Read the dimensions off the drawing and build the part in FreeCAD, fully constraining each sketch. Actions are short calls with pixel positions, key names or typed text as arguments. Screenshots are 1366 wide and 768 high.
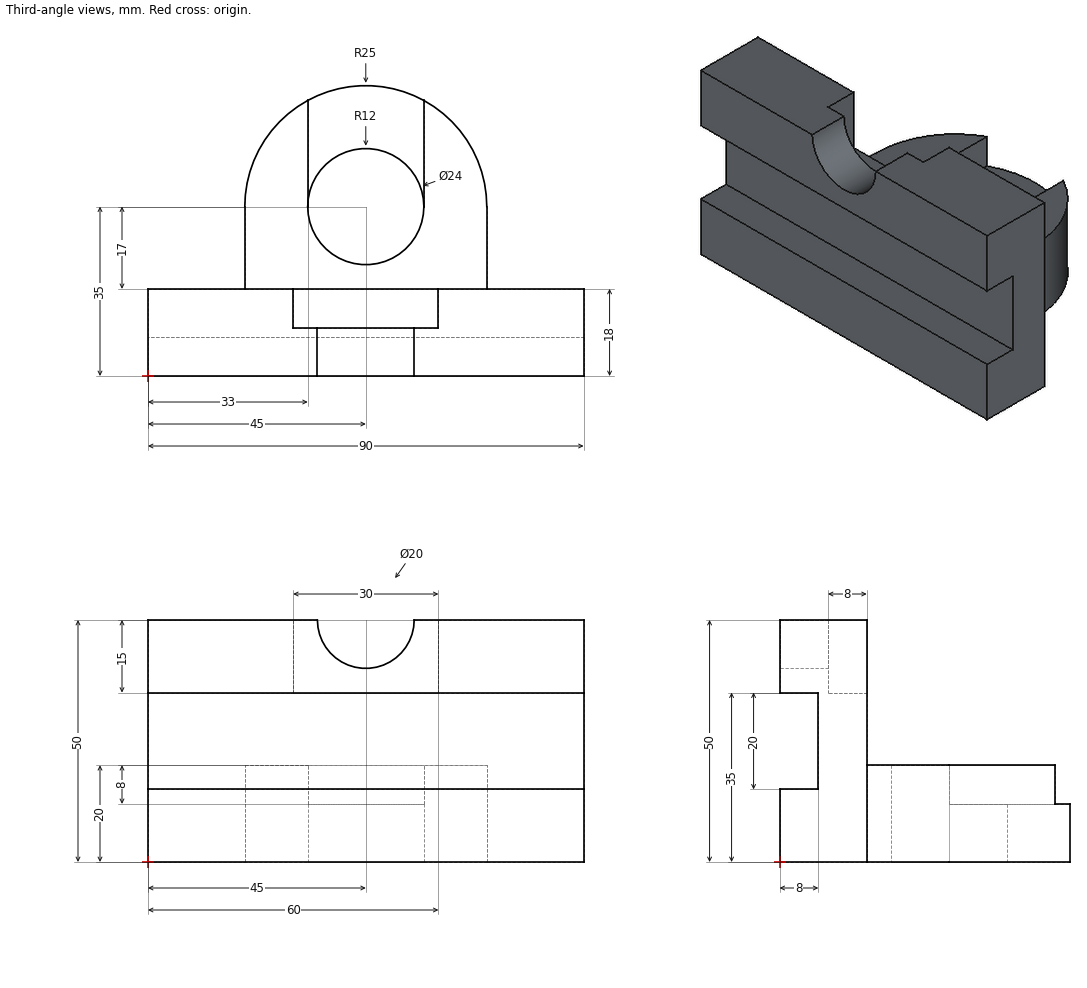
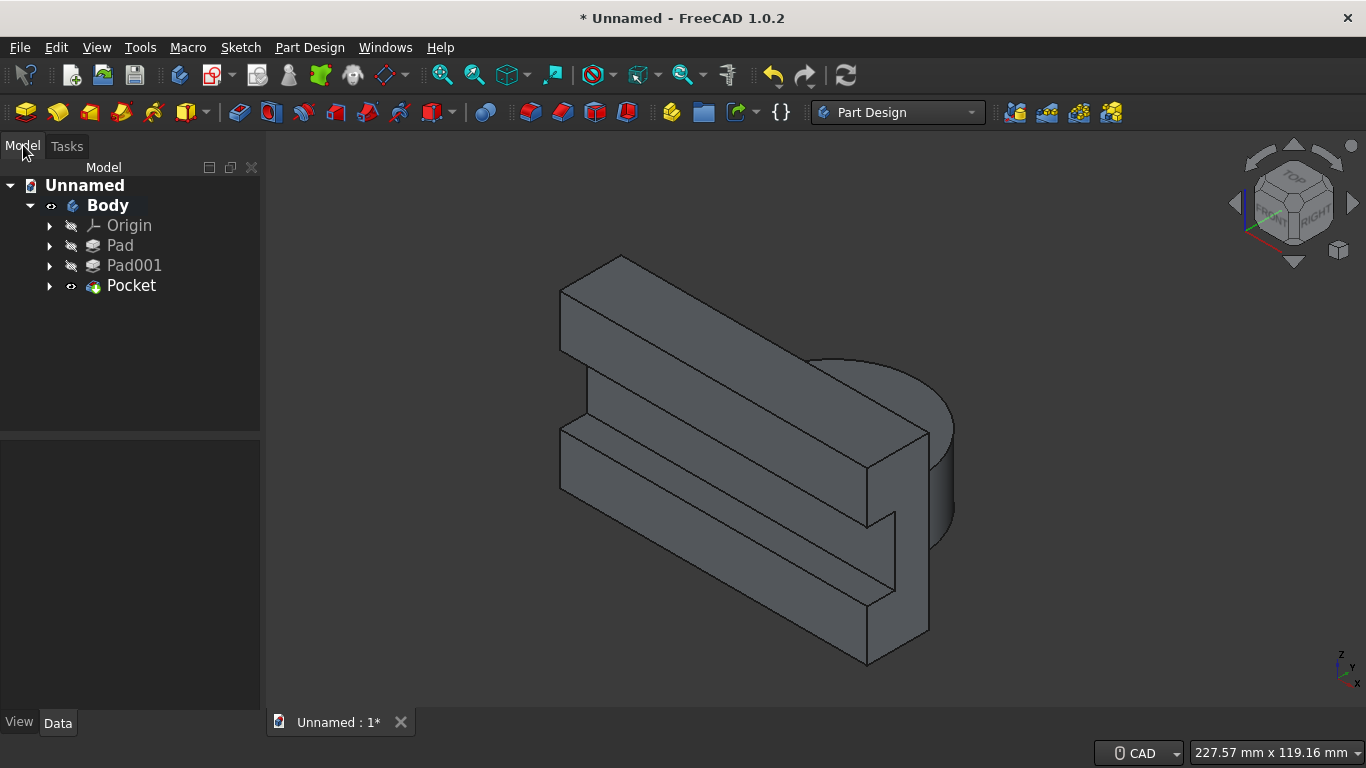
click(50, 226)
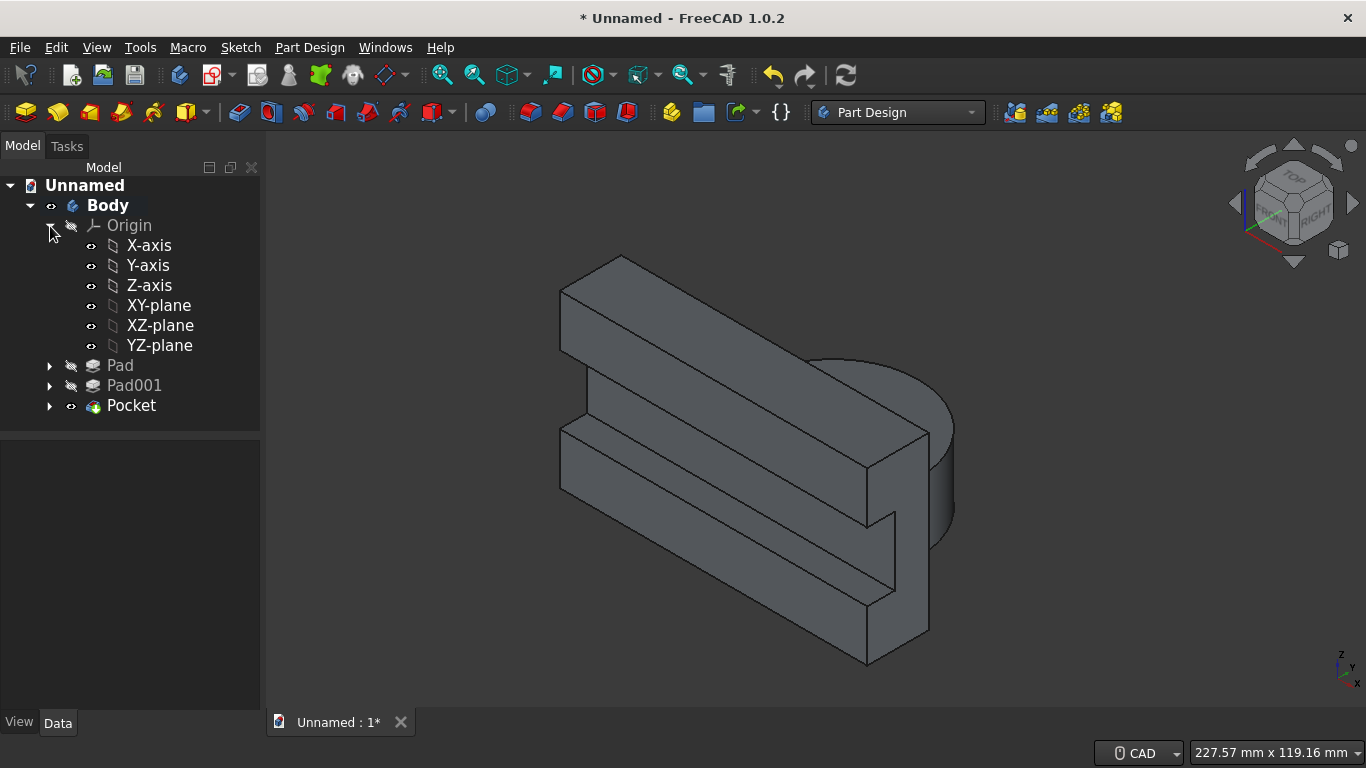
click(136, 306)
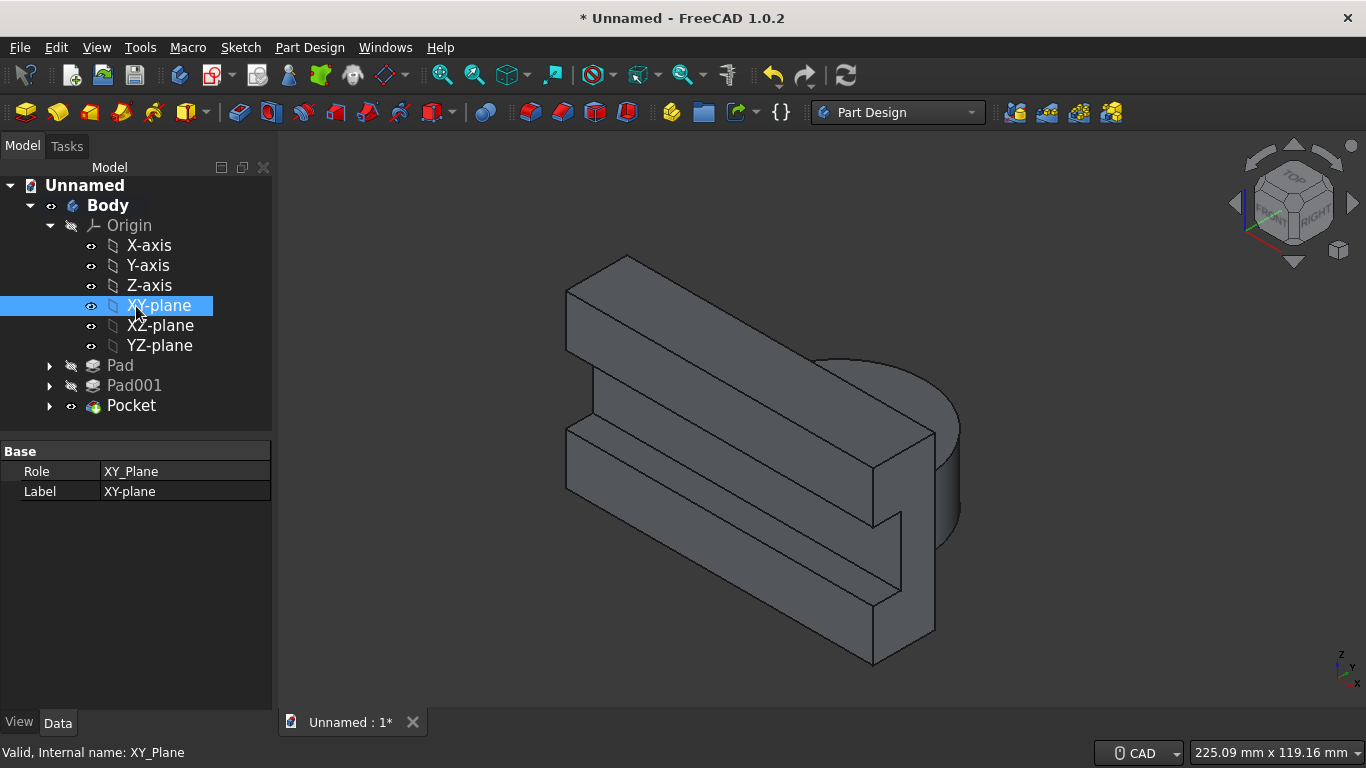
click(386, 76)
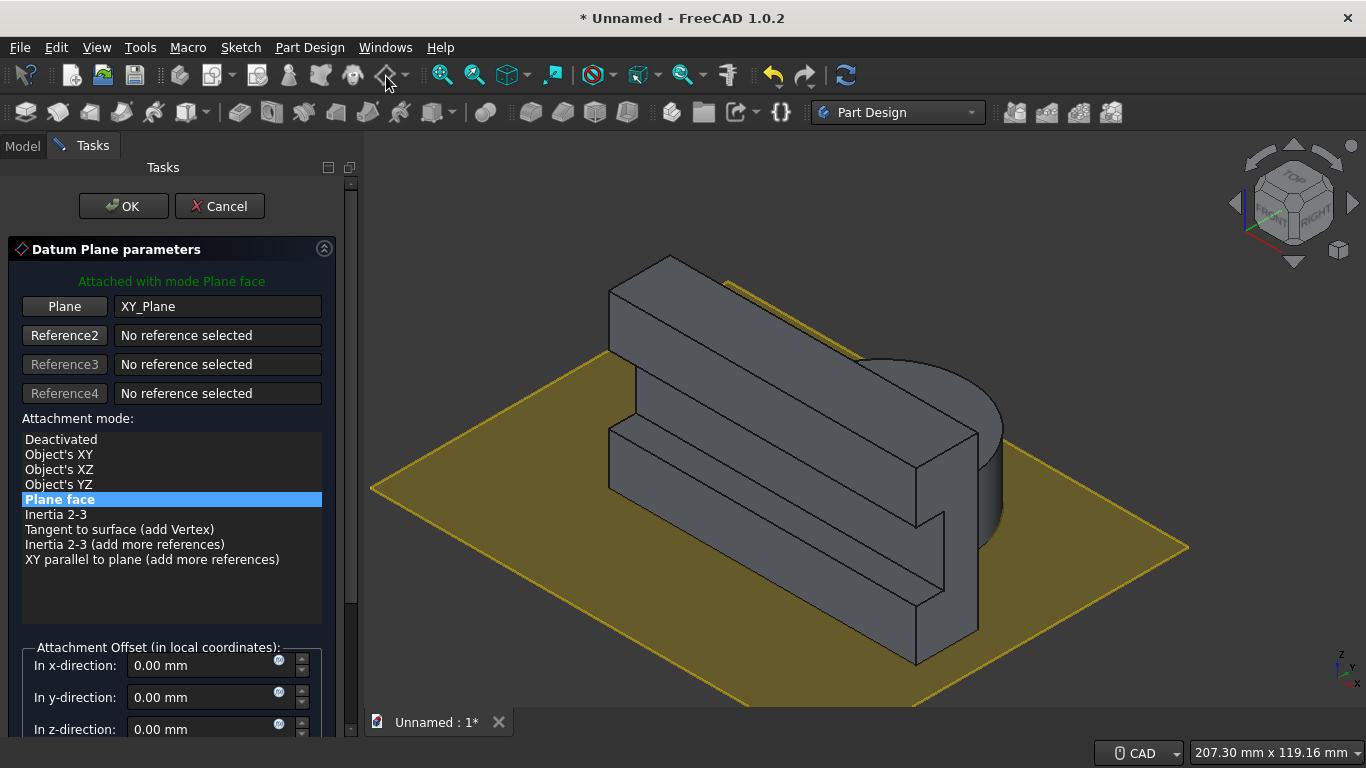
scroll(351, 456, down, 2)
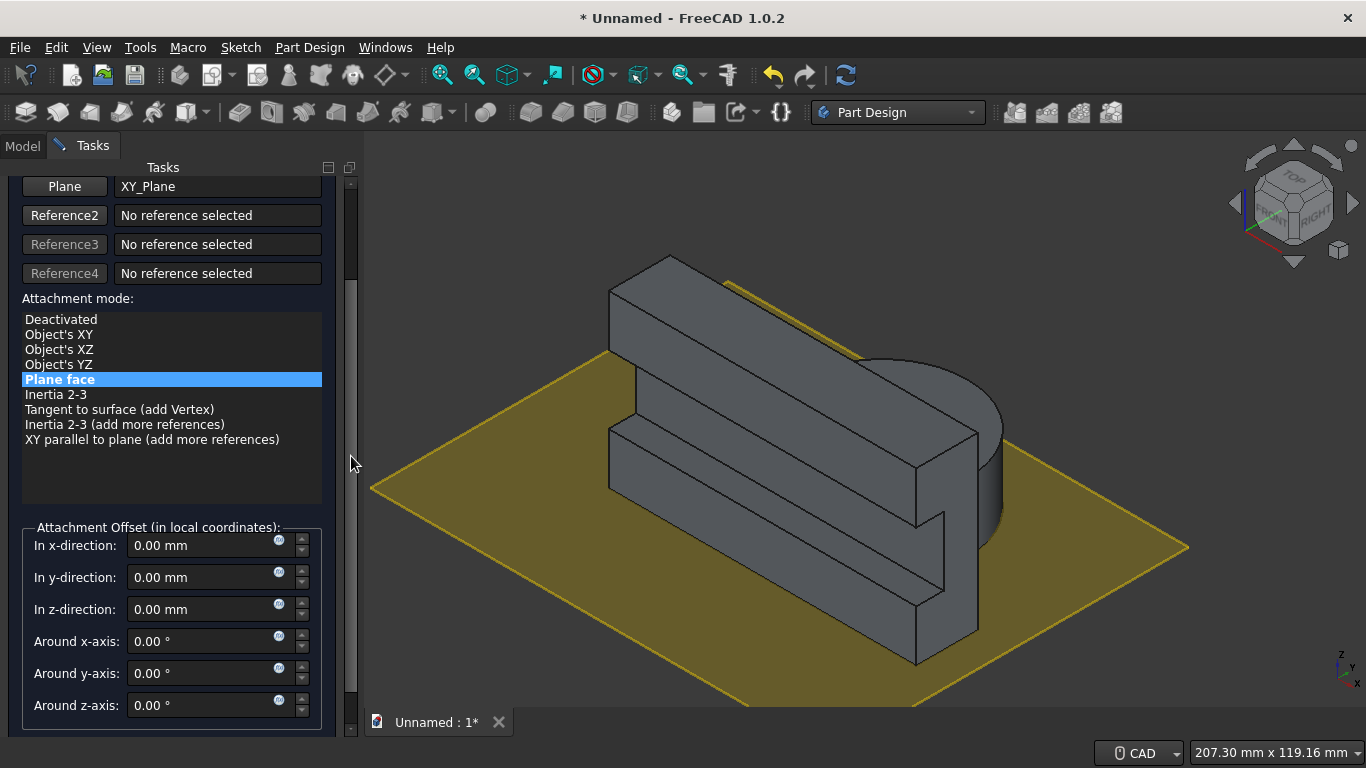
triple_click(210, 609)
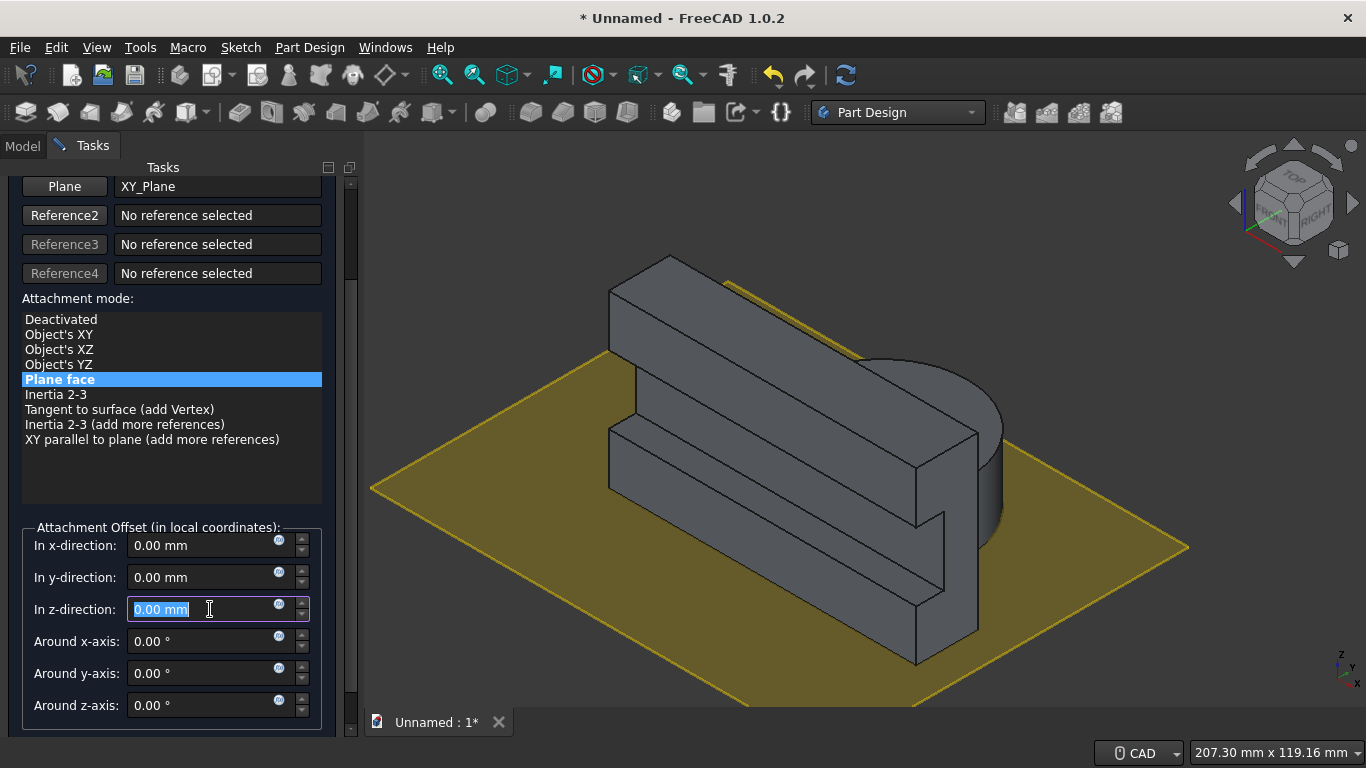
text(12)
key(Tab)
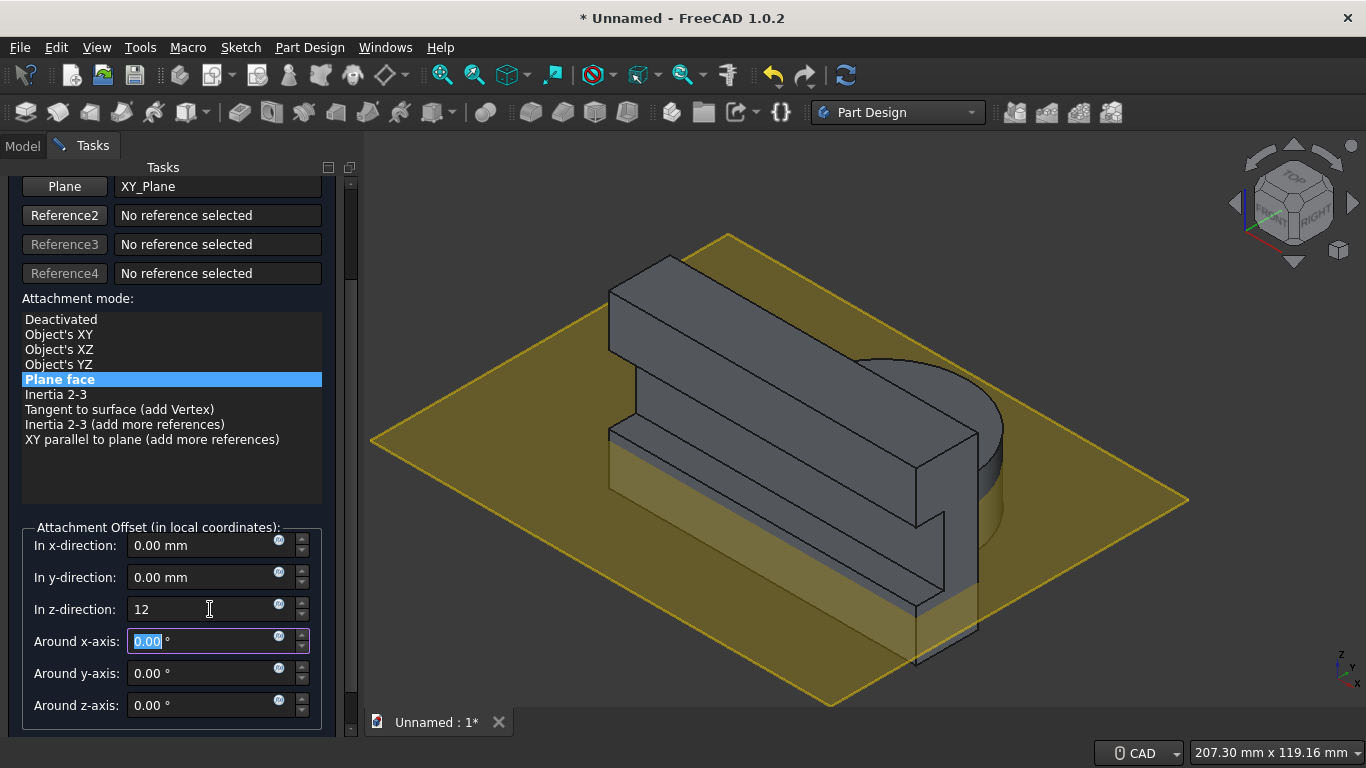
scroll(351, 456, up, 3)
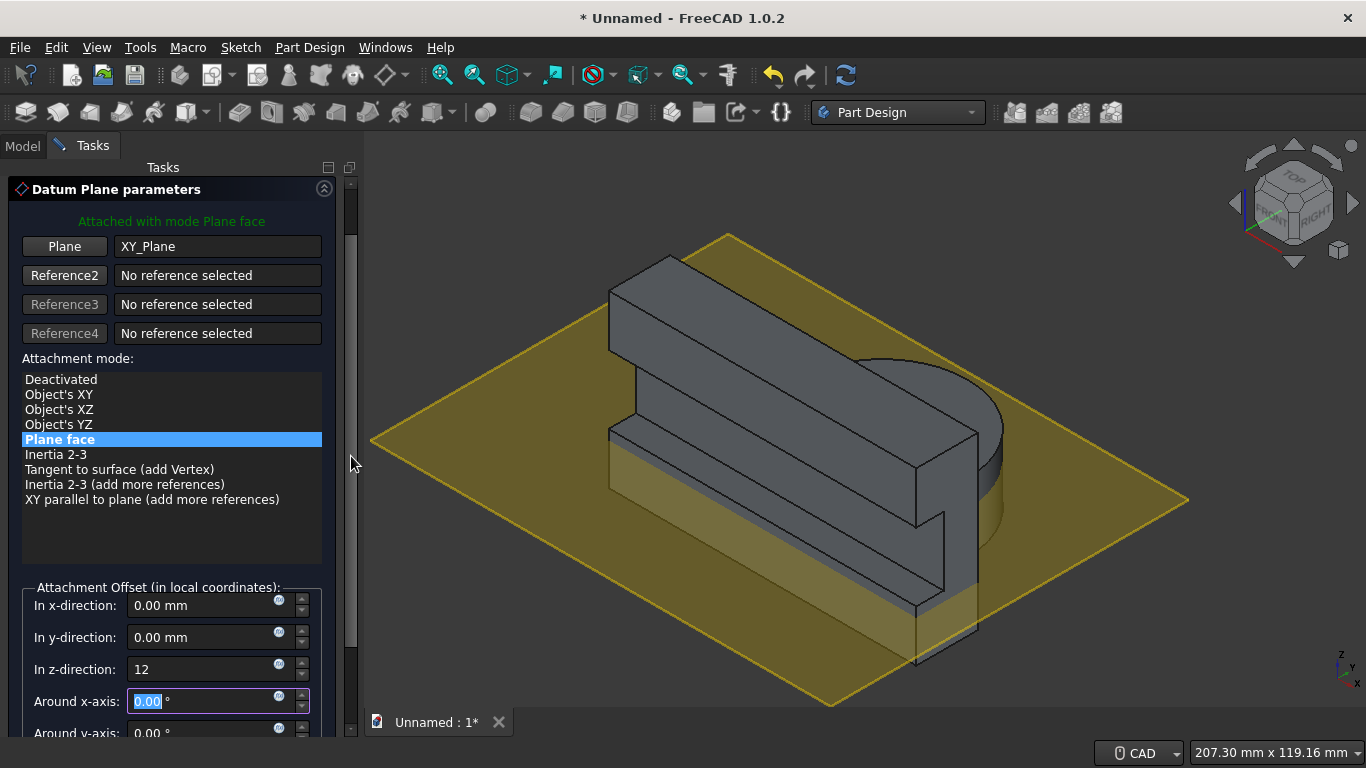
click(124, 206)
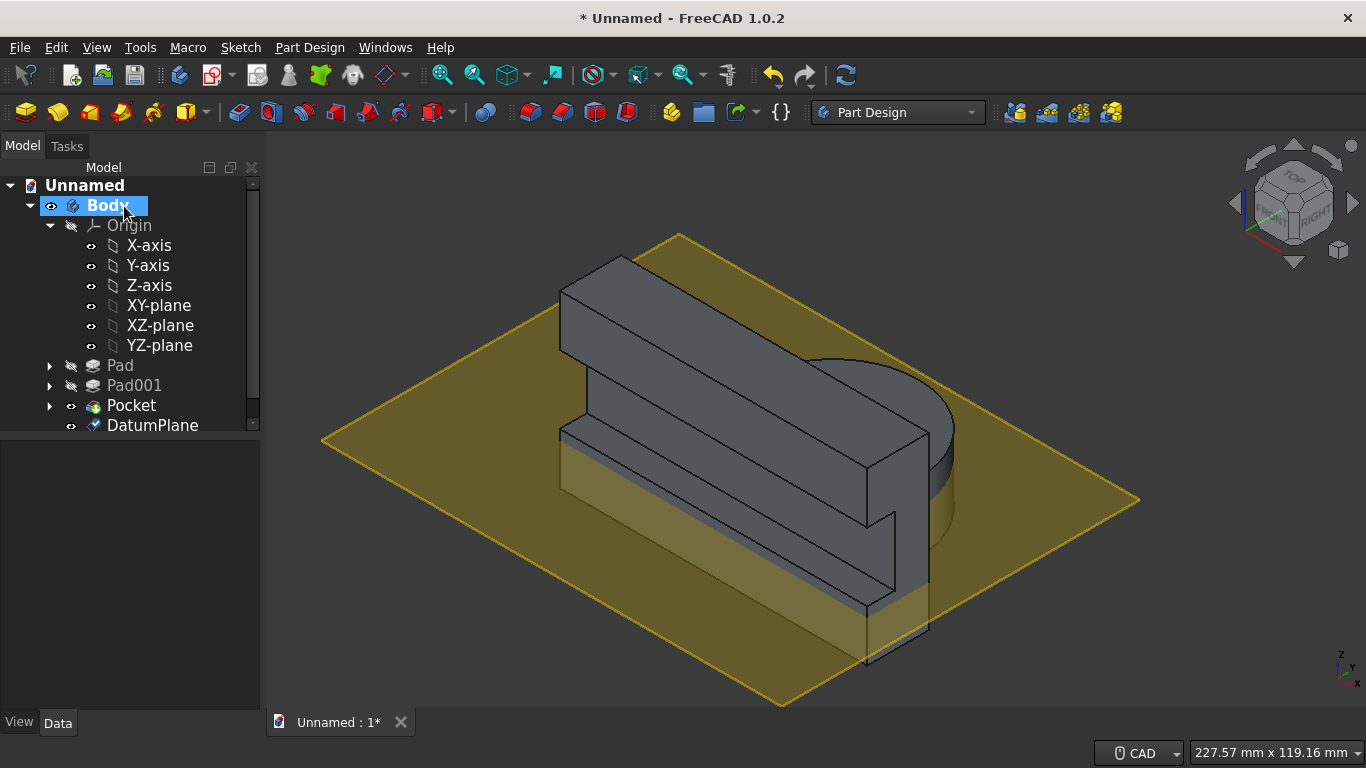
click(116, 426)